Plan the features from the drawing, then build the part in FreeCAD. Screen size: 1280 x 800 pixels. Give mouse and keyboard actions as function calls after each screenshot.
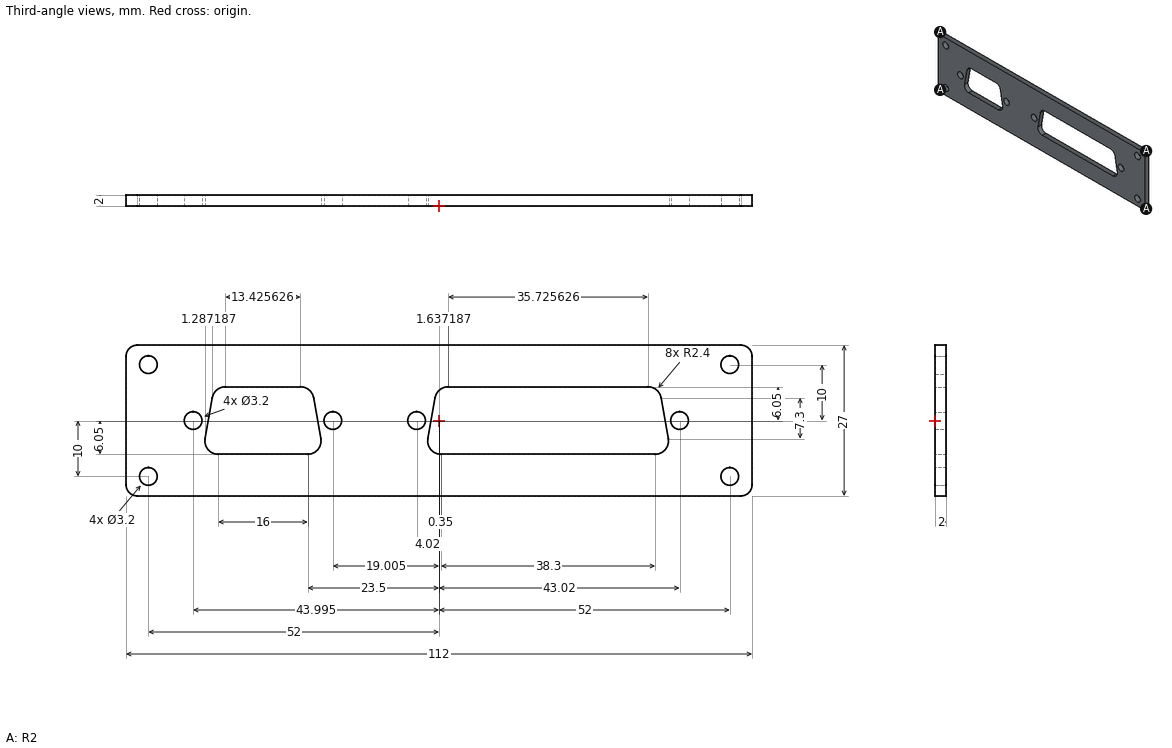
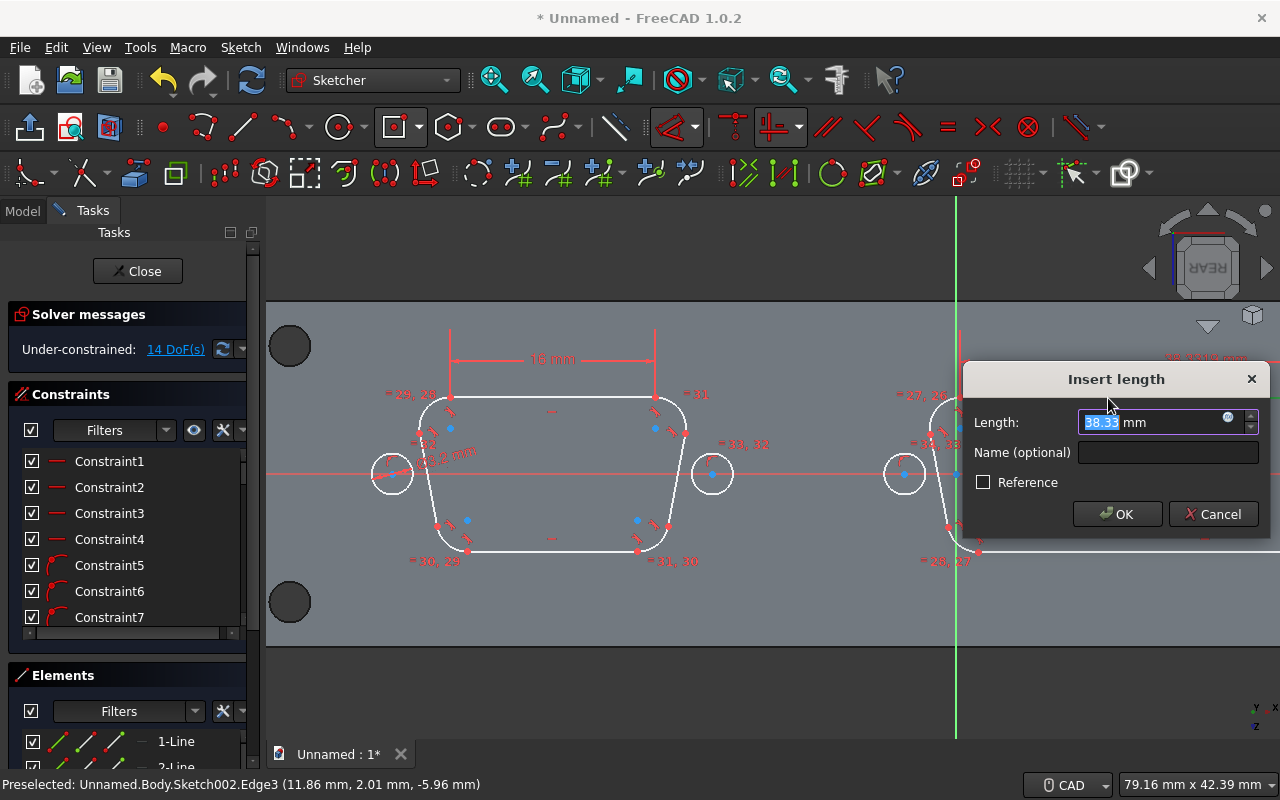
text(38.3)
key(Return)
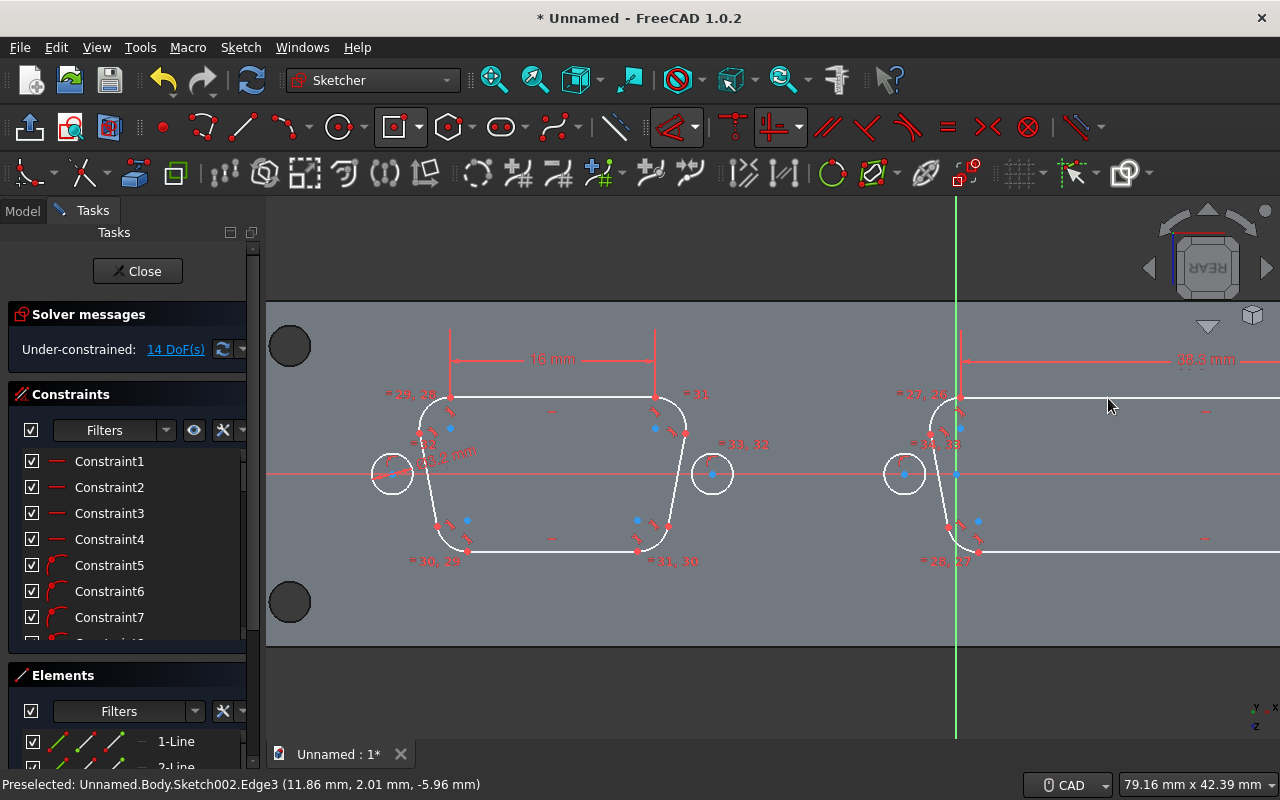
scroll(406, 460, down, 3)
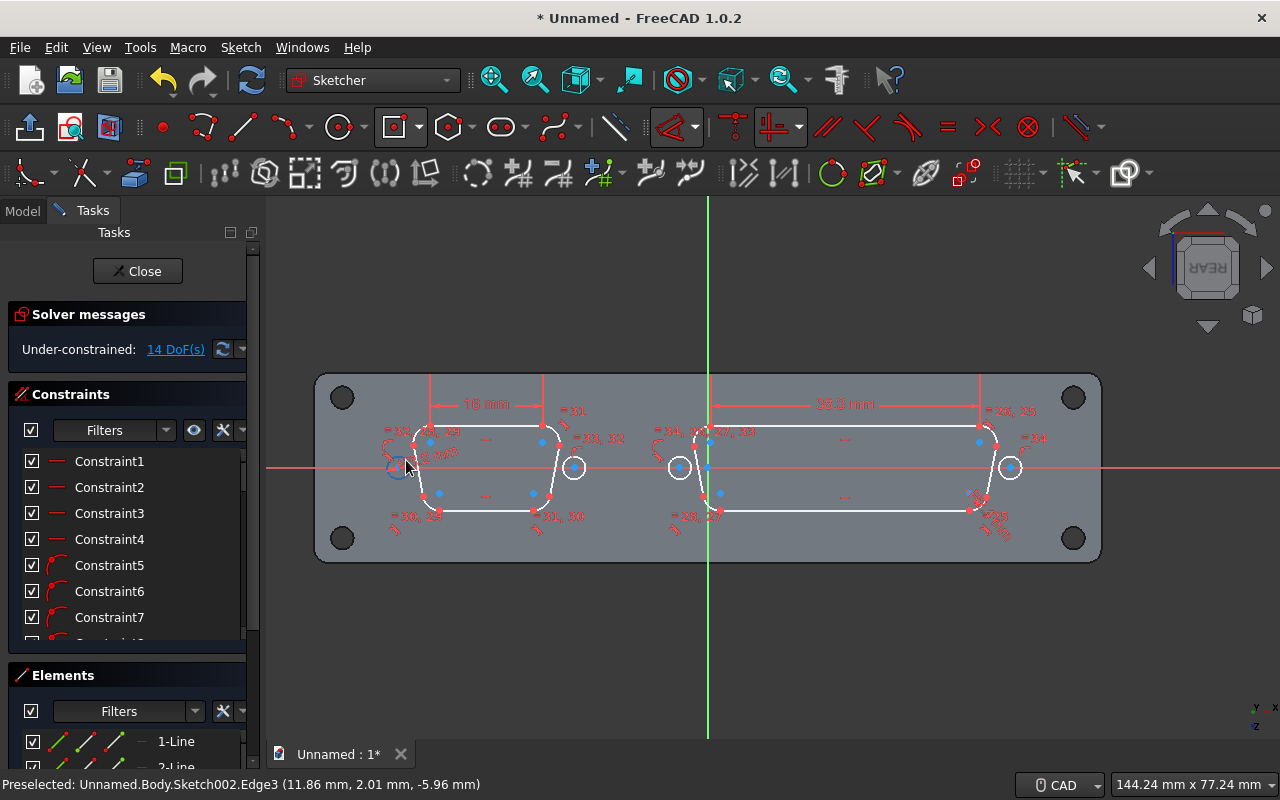
click(990, 482)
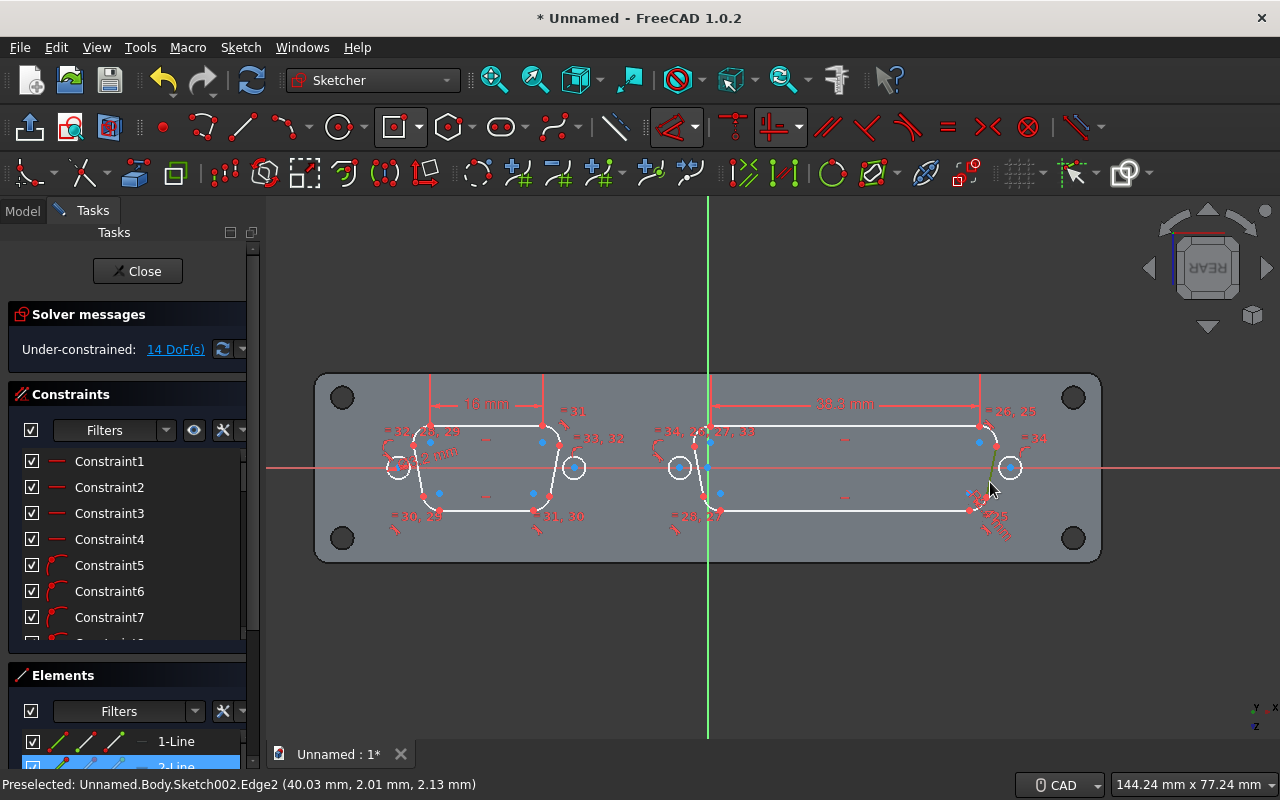
click(698, 128)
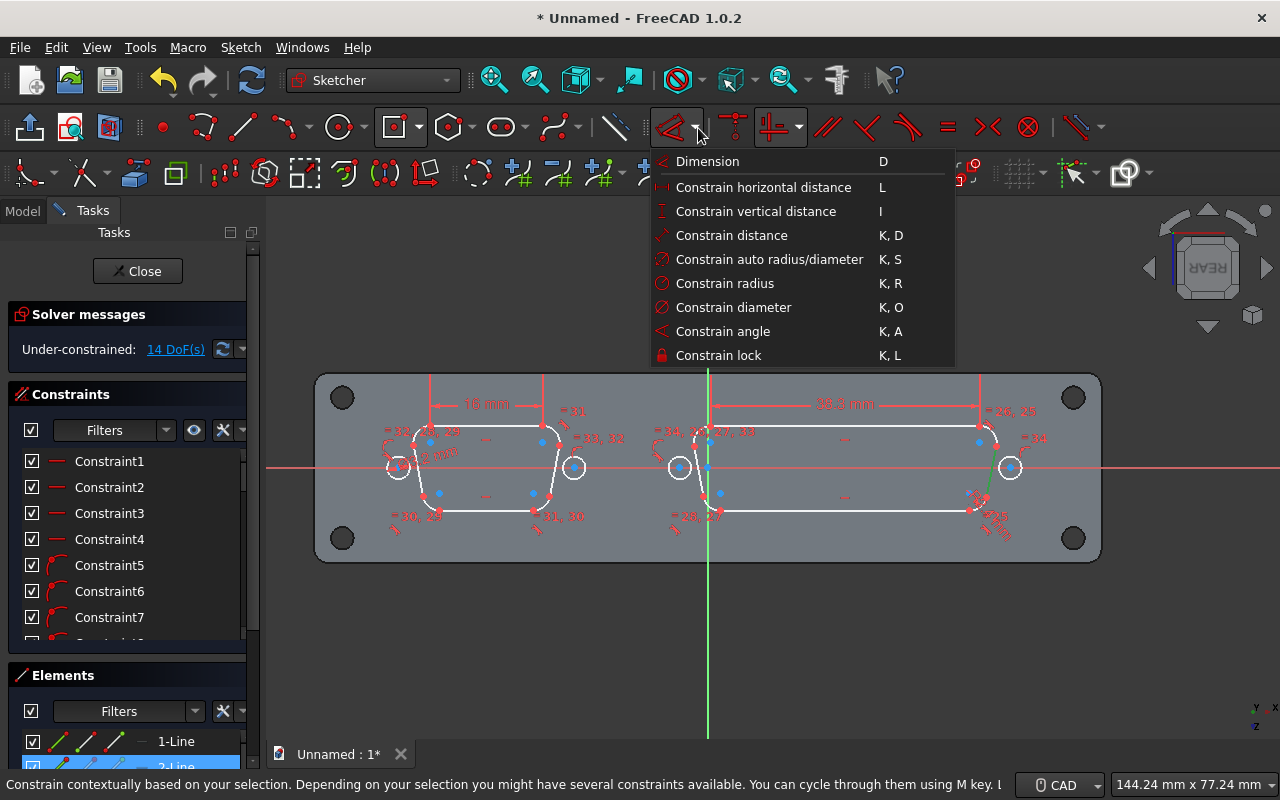
click(803, 211)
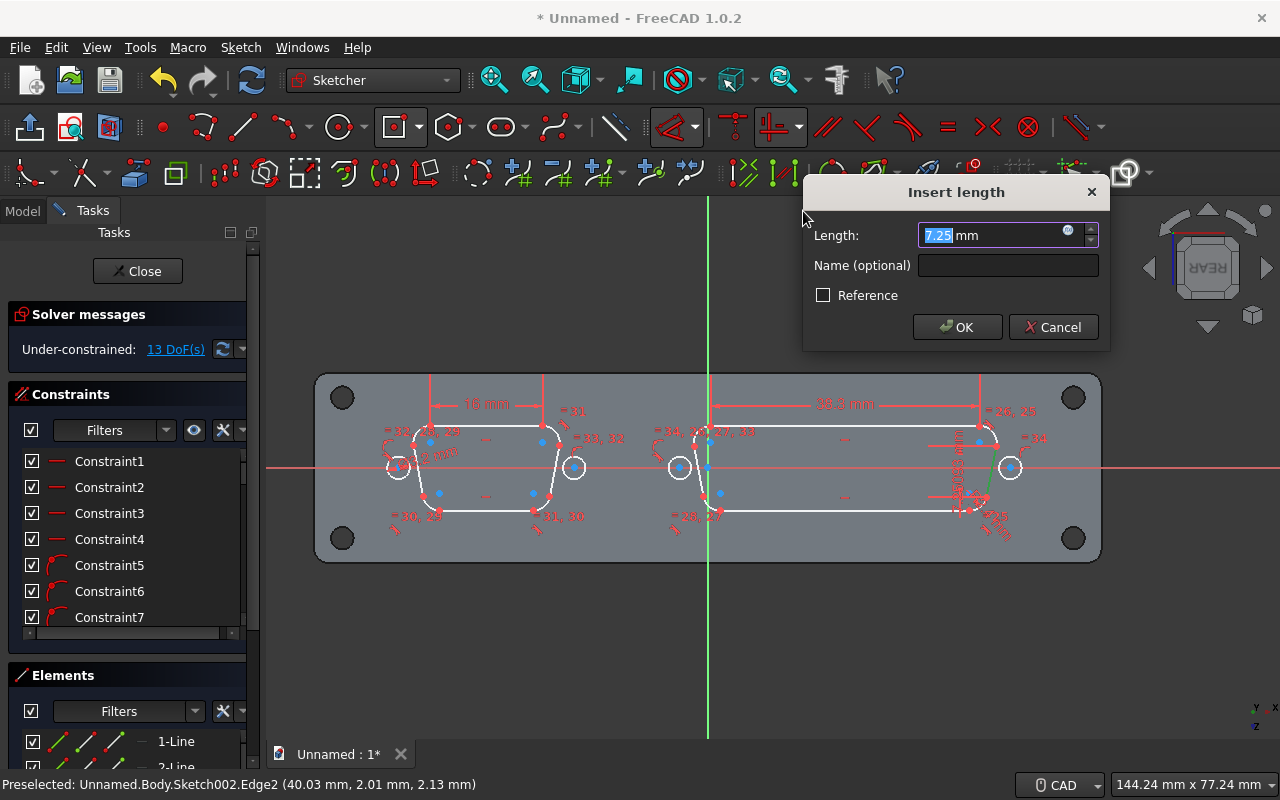
text(7.3)
key(Return)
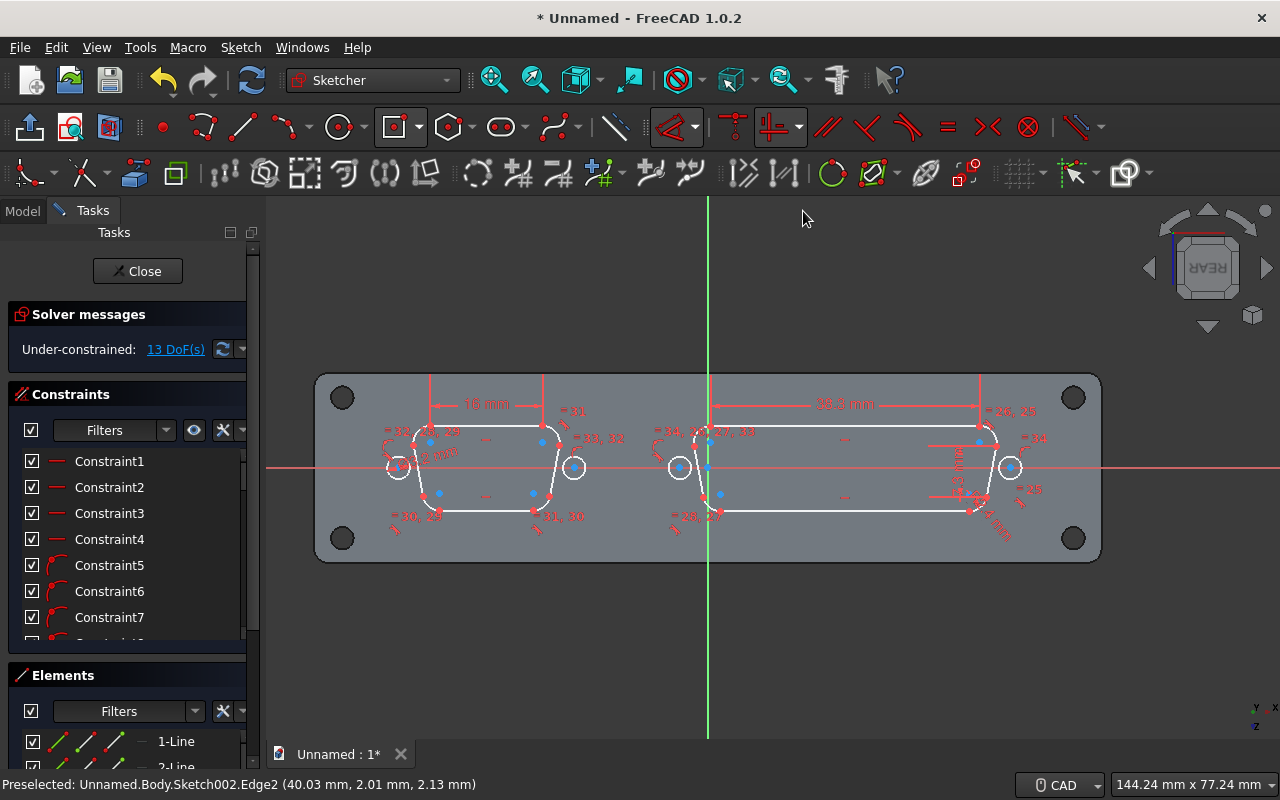
click(420, 481)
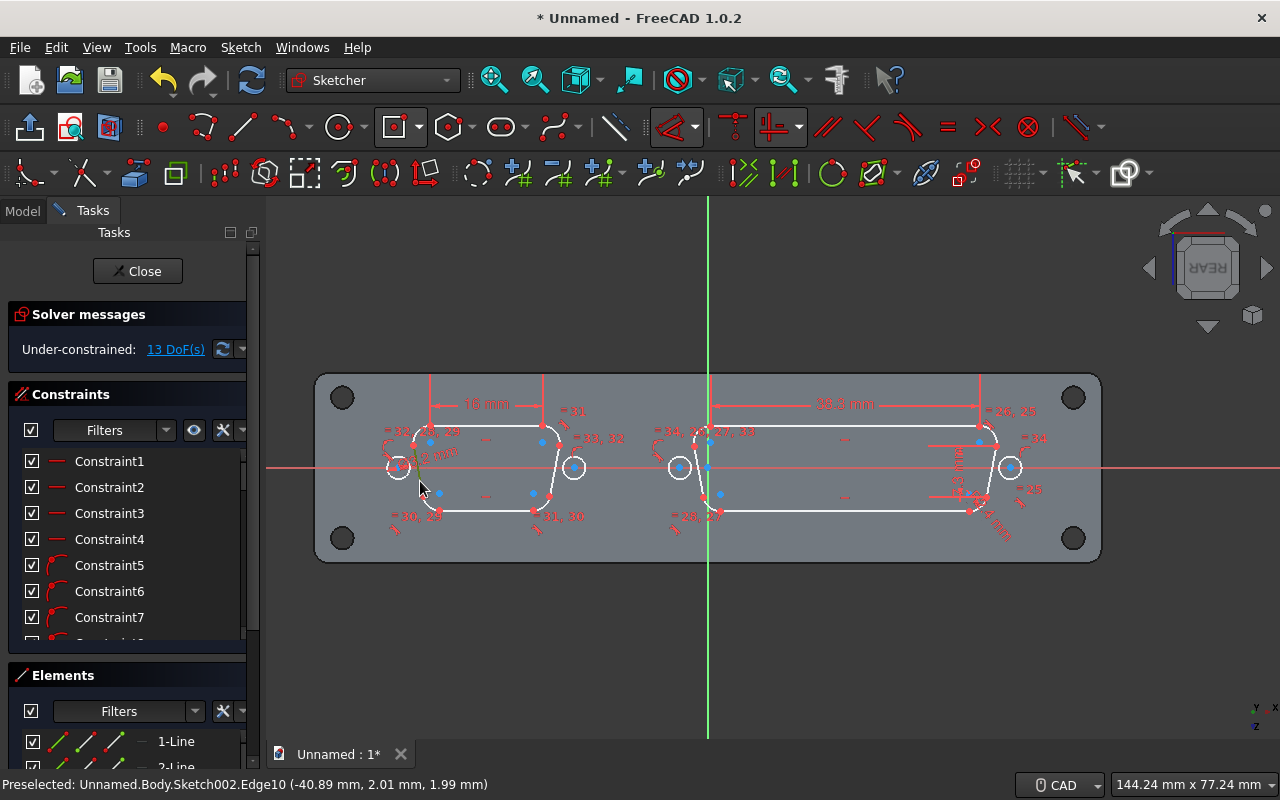
key(i)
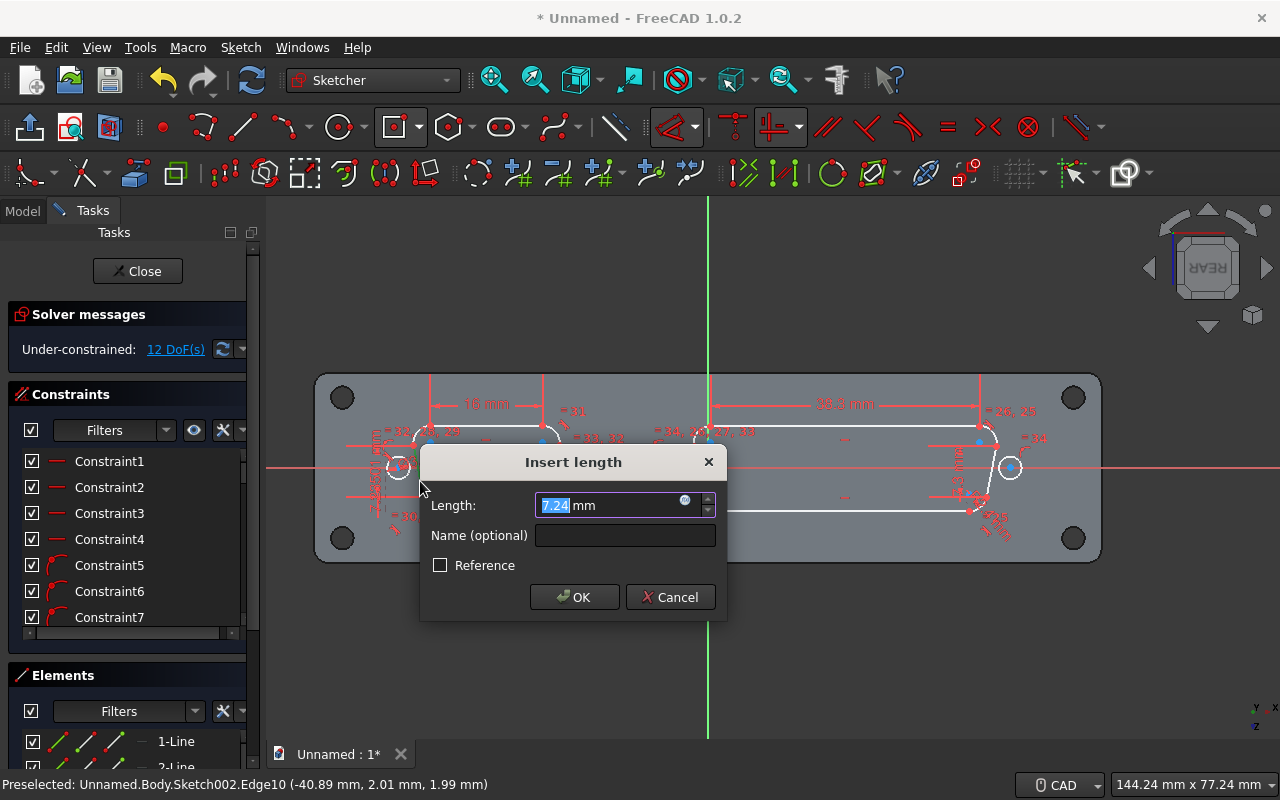
text(7.3)
key(Return)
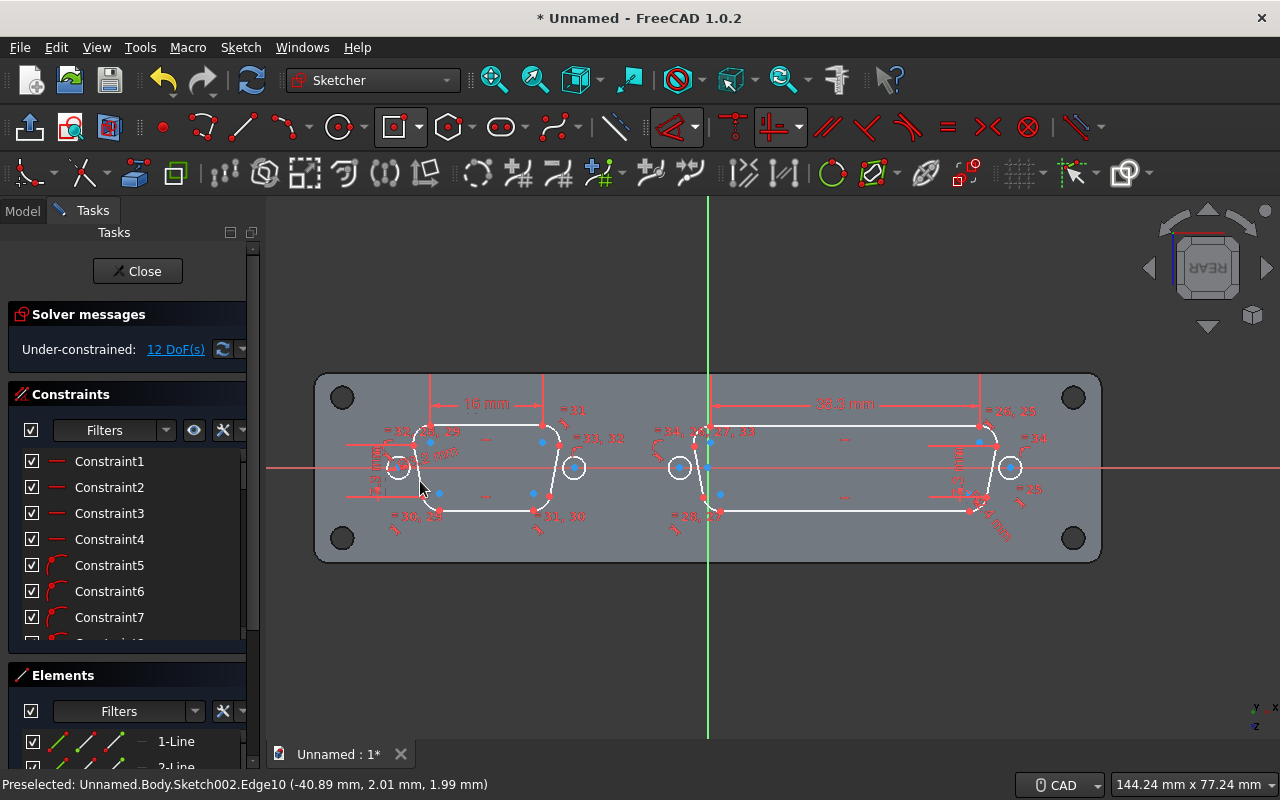
scroll(680, 468, up, 2)